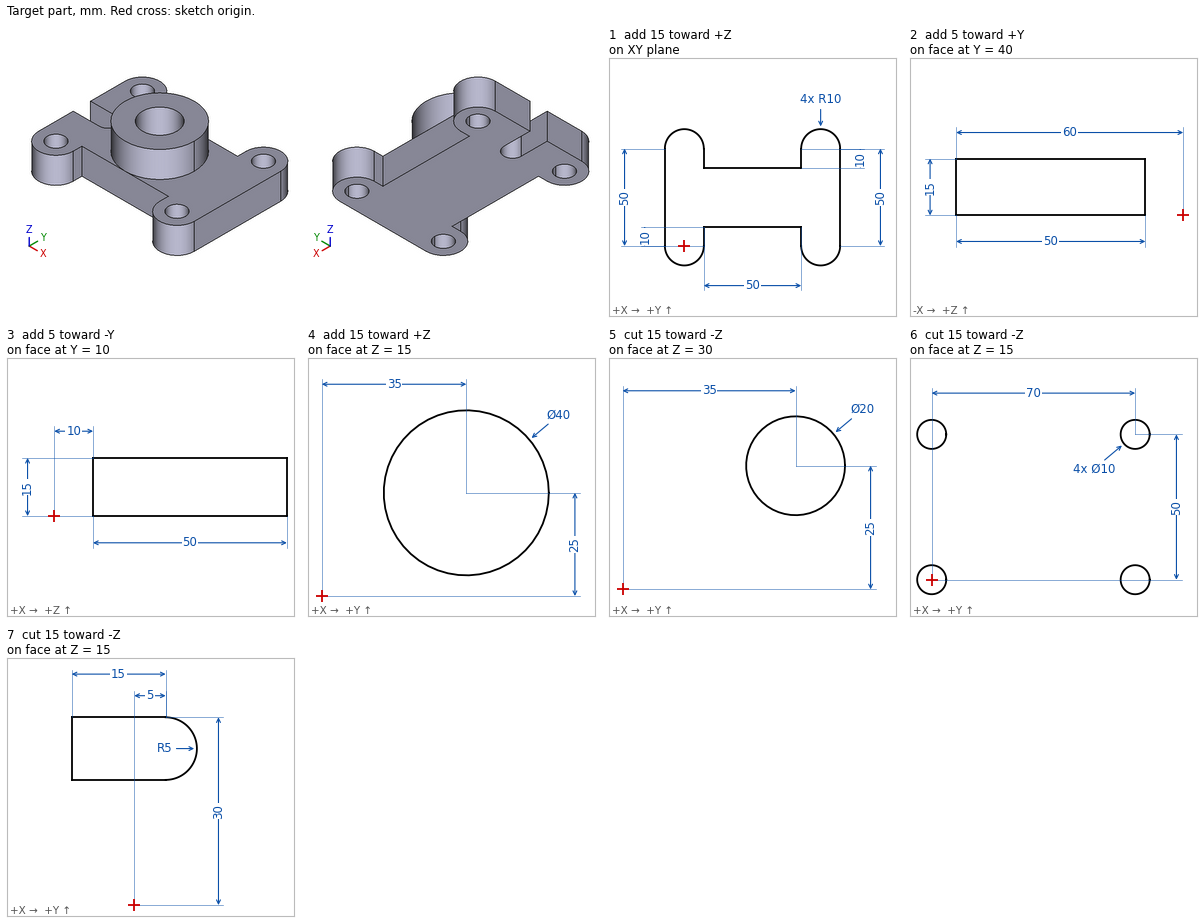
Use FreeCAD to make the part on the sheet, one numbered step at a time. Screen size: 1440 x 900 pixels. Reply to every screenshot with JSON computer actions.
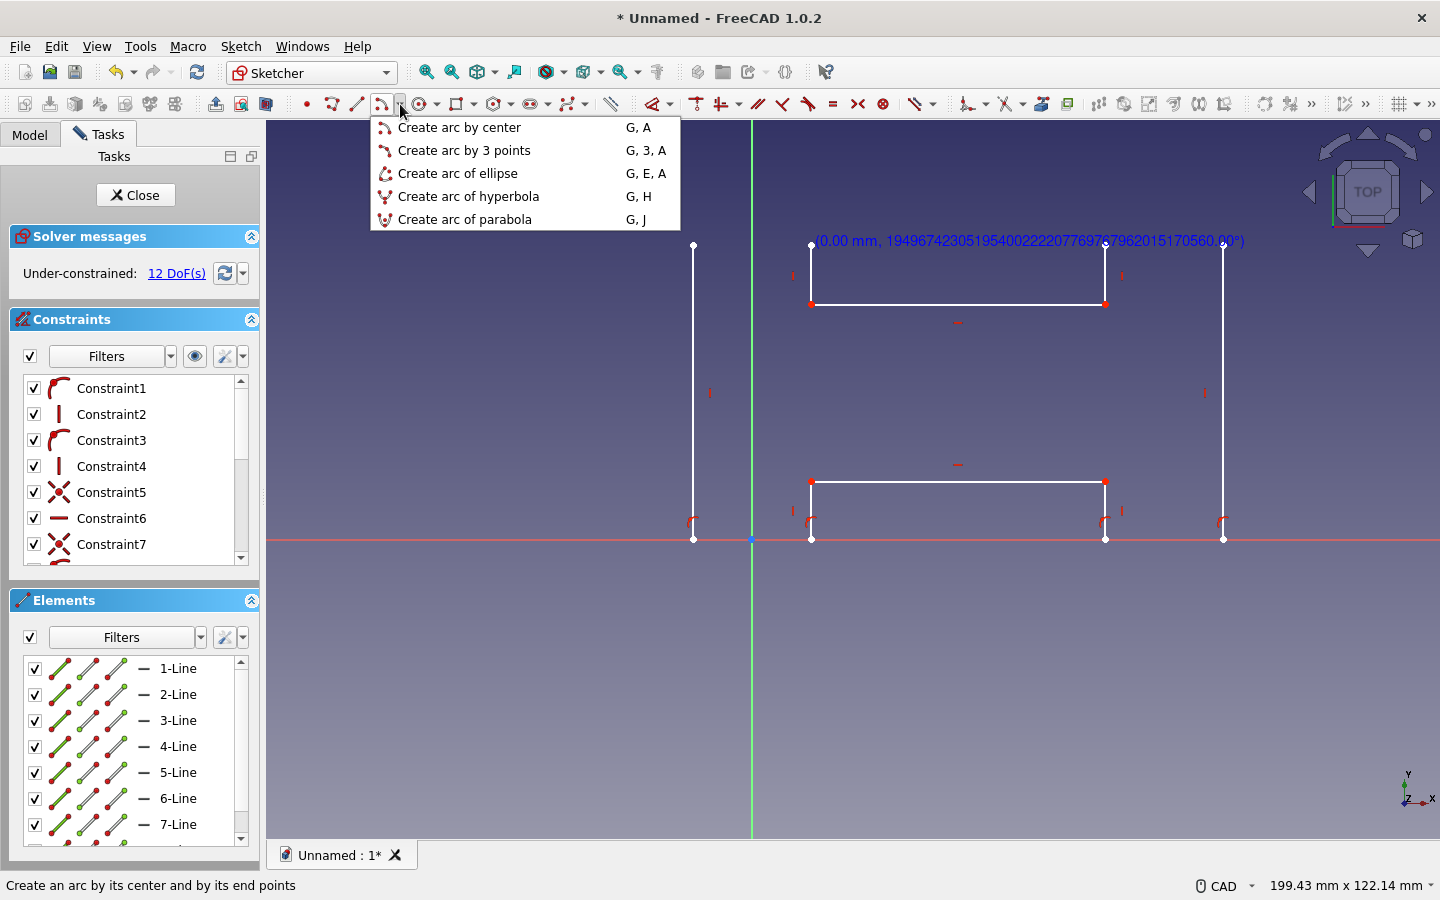
{"action": "left_click", "coordinate": [526, 150]}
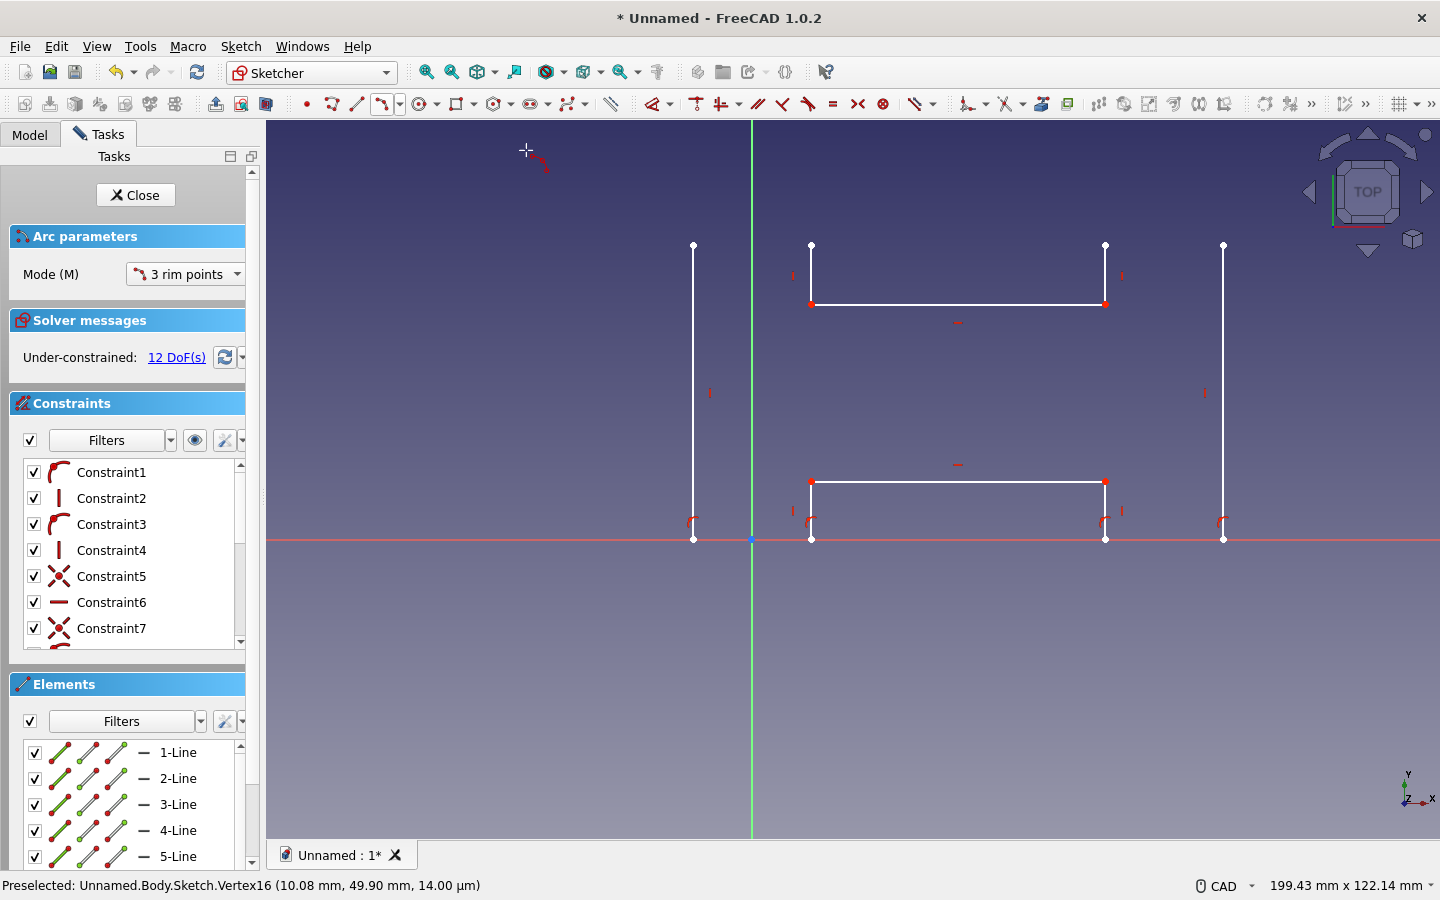
{"action": "left_click", "coordinate": [693, 540]}
{"action": "left_click", "coordinate": [811, 540]}
{"action": "left_click", "coordinate": [733, 596]}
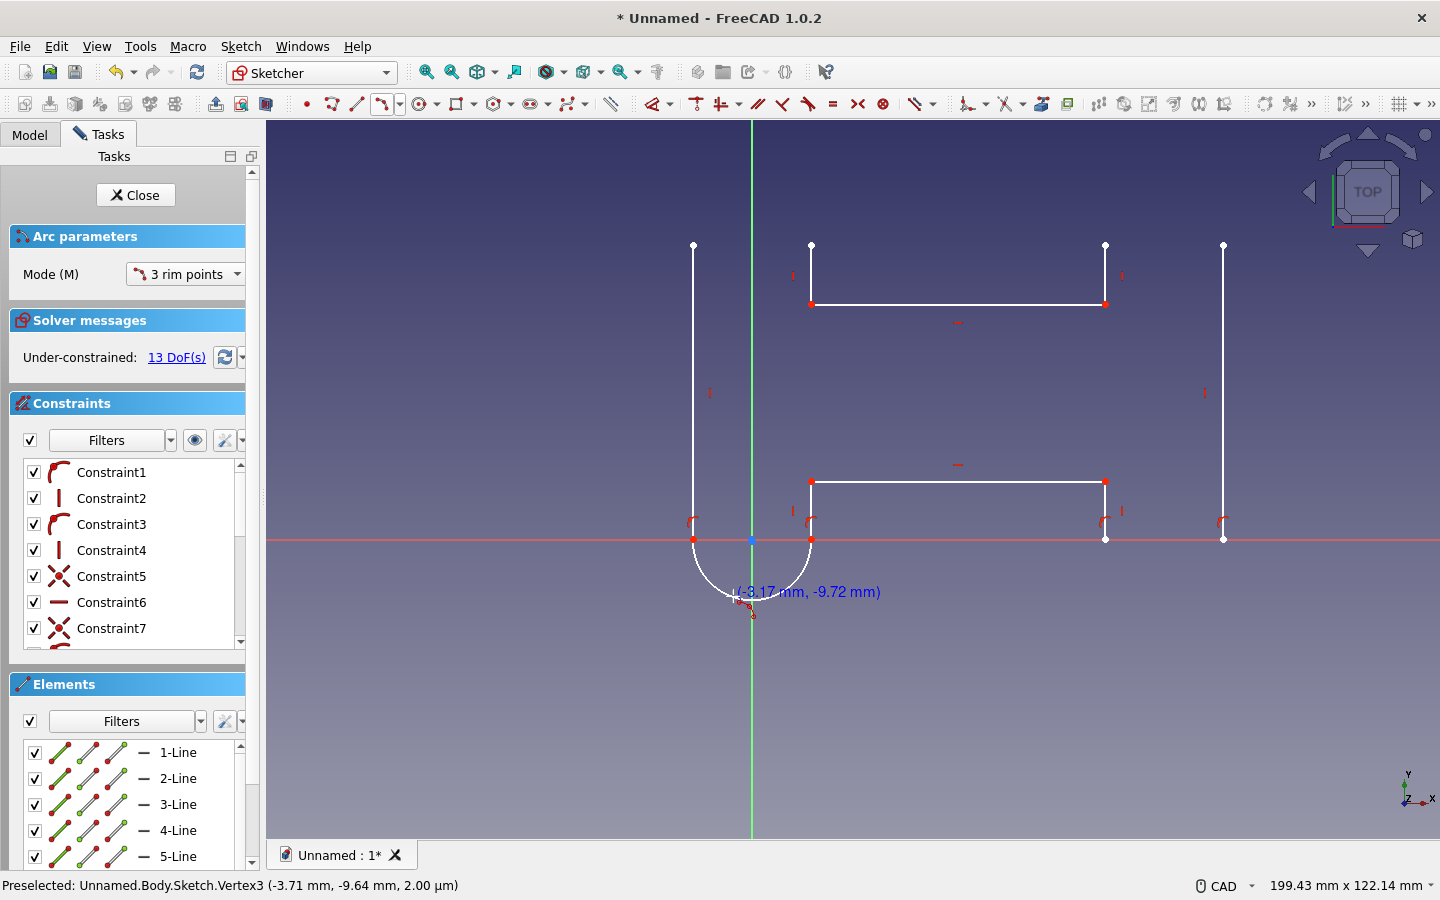
{"action": "left_click", "coordinate": [1105, 540]}
{"action": "left_click", "coordinate": [1223, 540]}
{"action": "left_click", "coordinate": [1164, 599]}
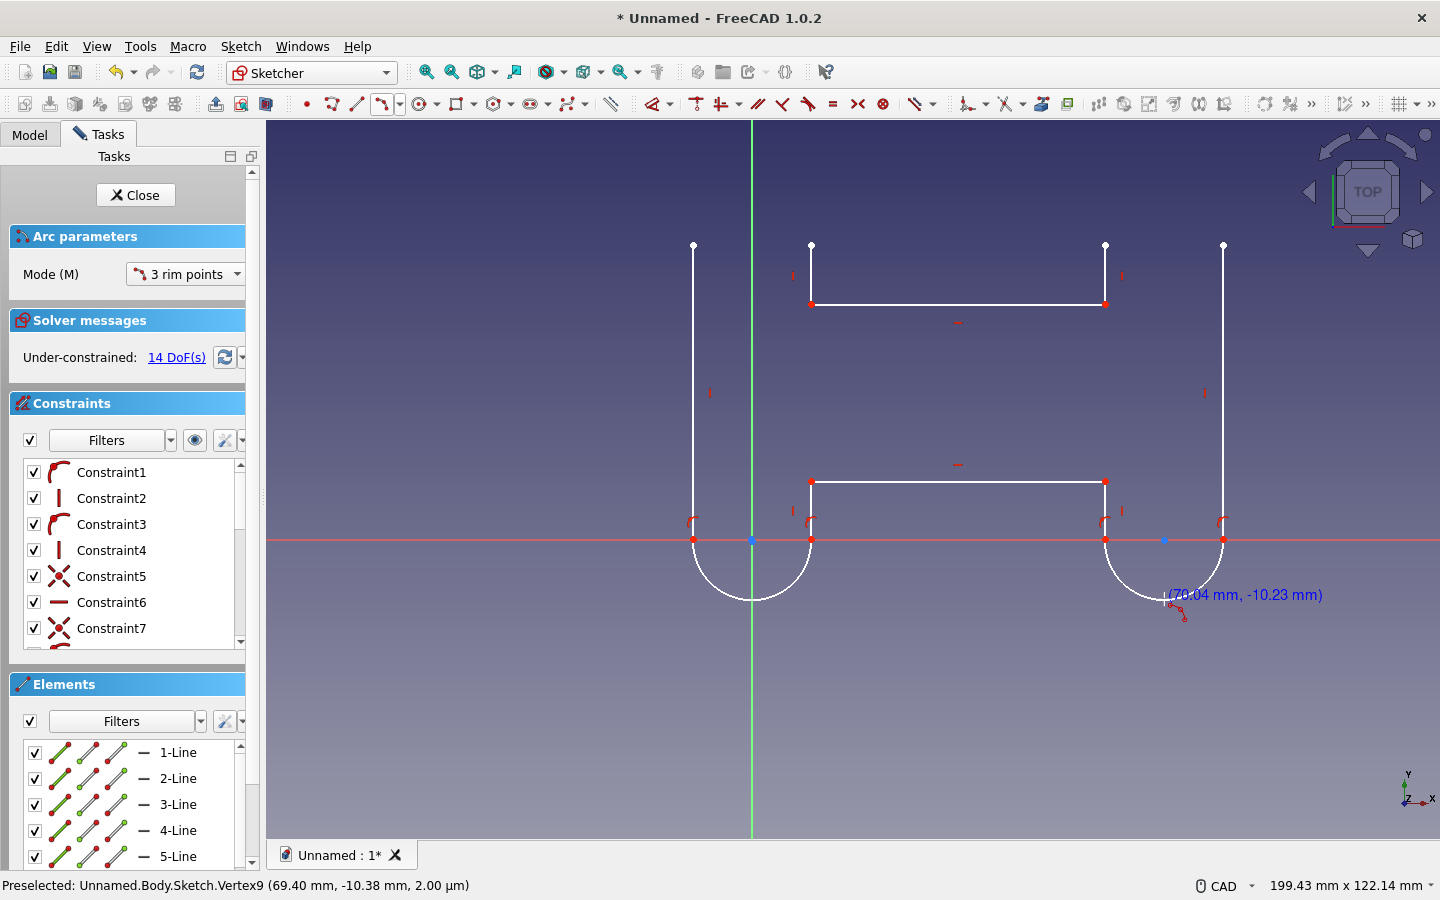
{"action": "left_click", "coordinate": [1223, 246]}
{"action": "left_click", "coordinate": [1105, 246]}
{"action": "left_click", "coordinate": [1164, 187]}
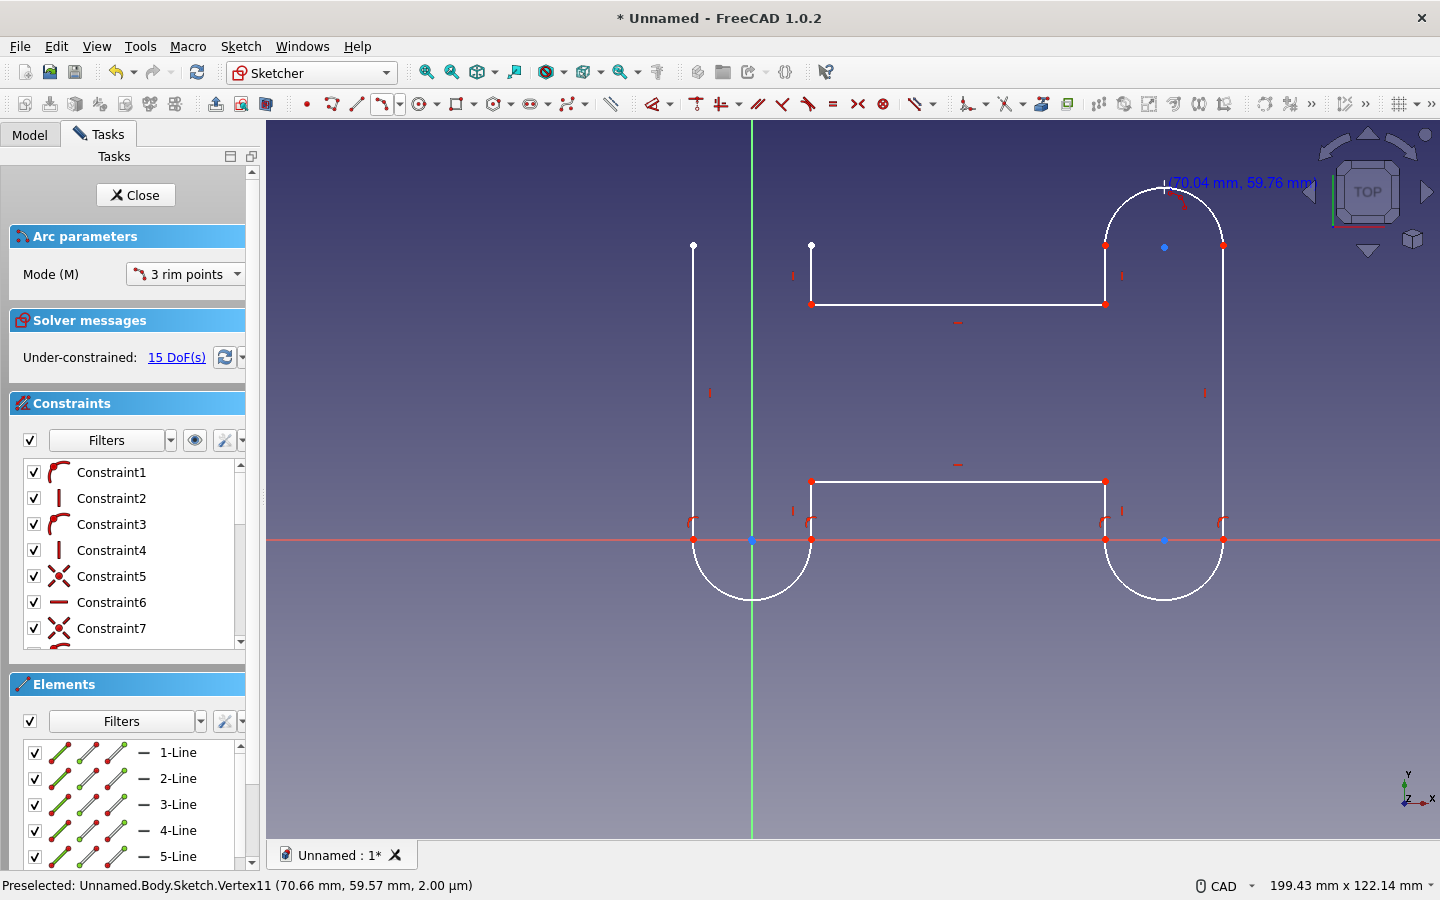
{"action": "left_click", "coordinate": [811, 246]}
{"action": "left_click", "coordinate": [693, 246]}
{"action": "left_click", "coordinate": [770, 189]}
{"action": "key", "text": "Escape"}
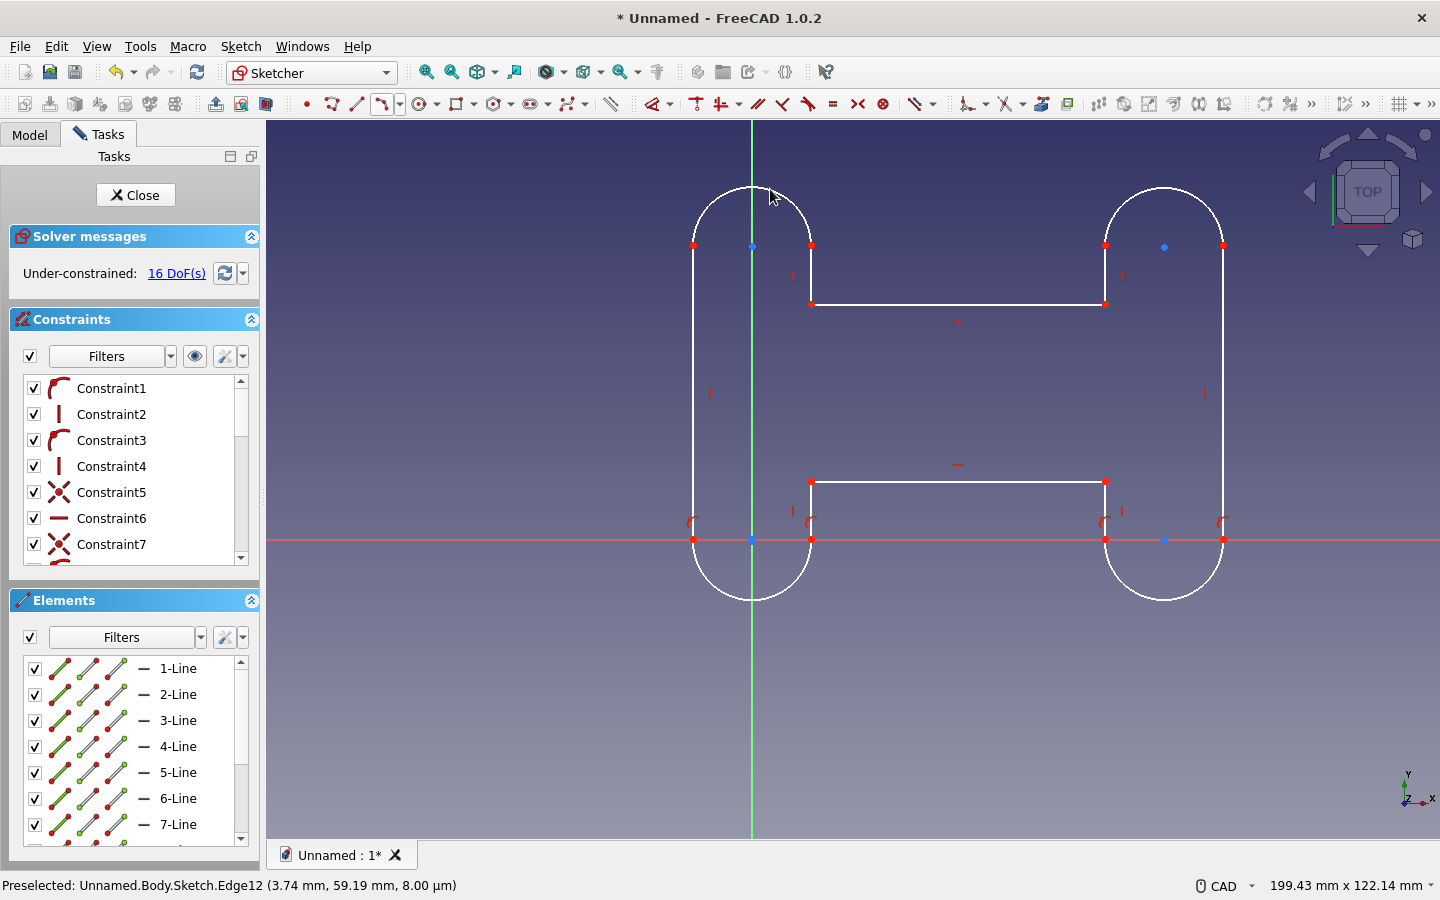
{"action": "left_click", "coordinate": [693, 334]}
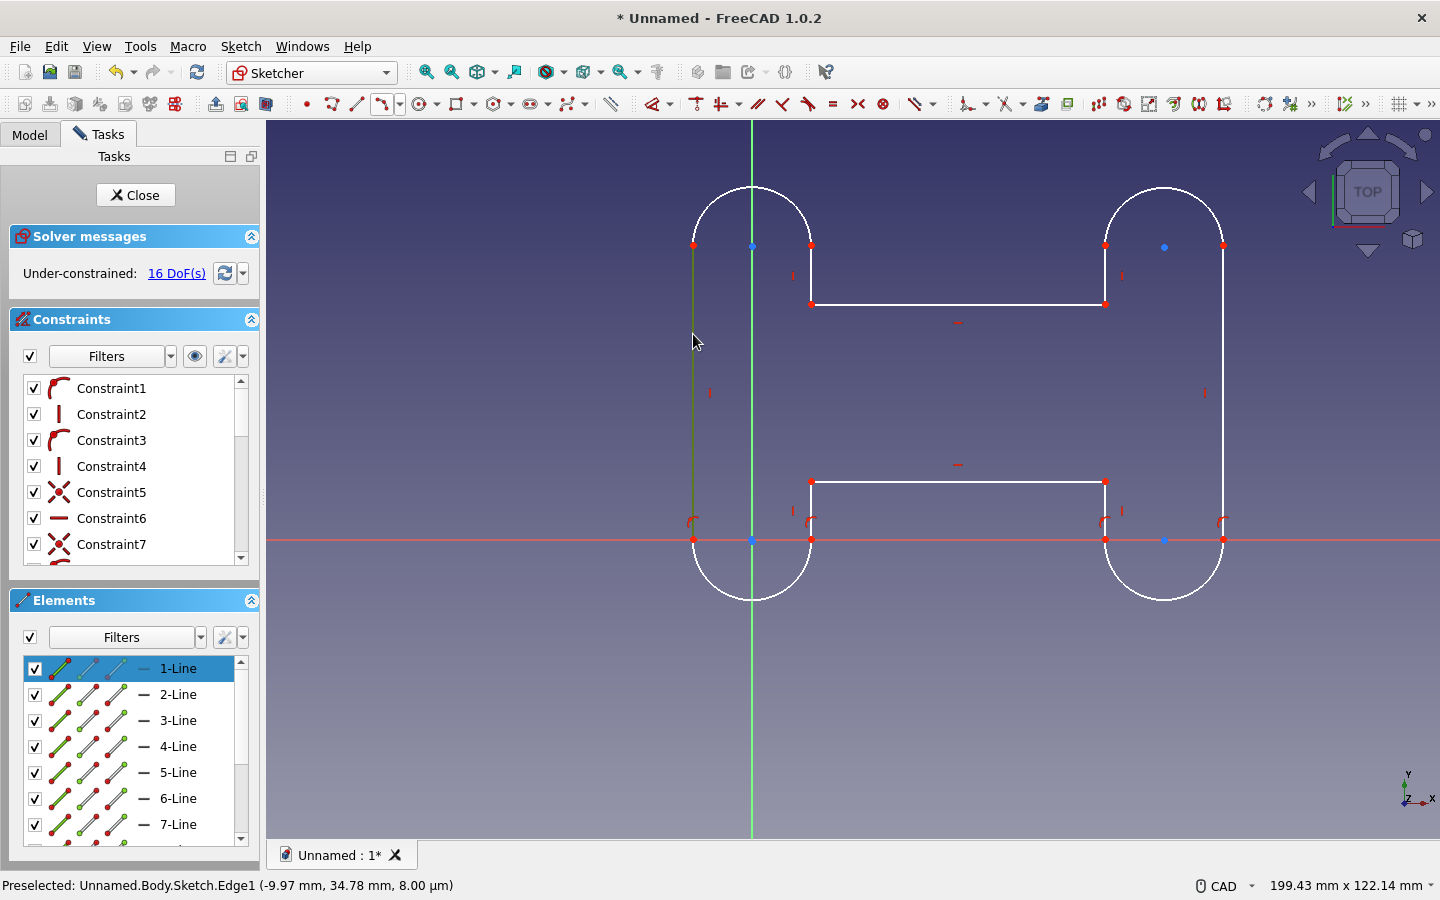
{"action": "left_click", "coordinate": [717, 589]}